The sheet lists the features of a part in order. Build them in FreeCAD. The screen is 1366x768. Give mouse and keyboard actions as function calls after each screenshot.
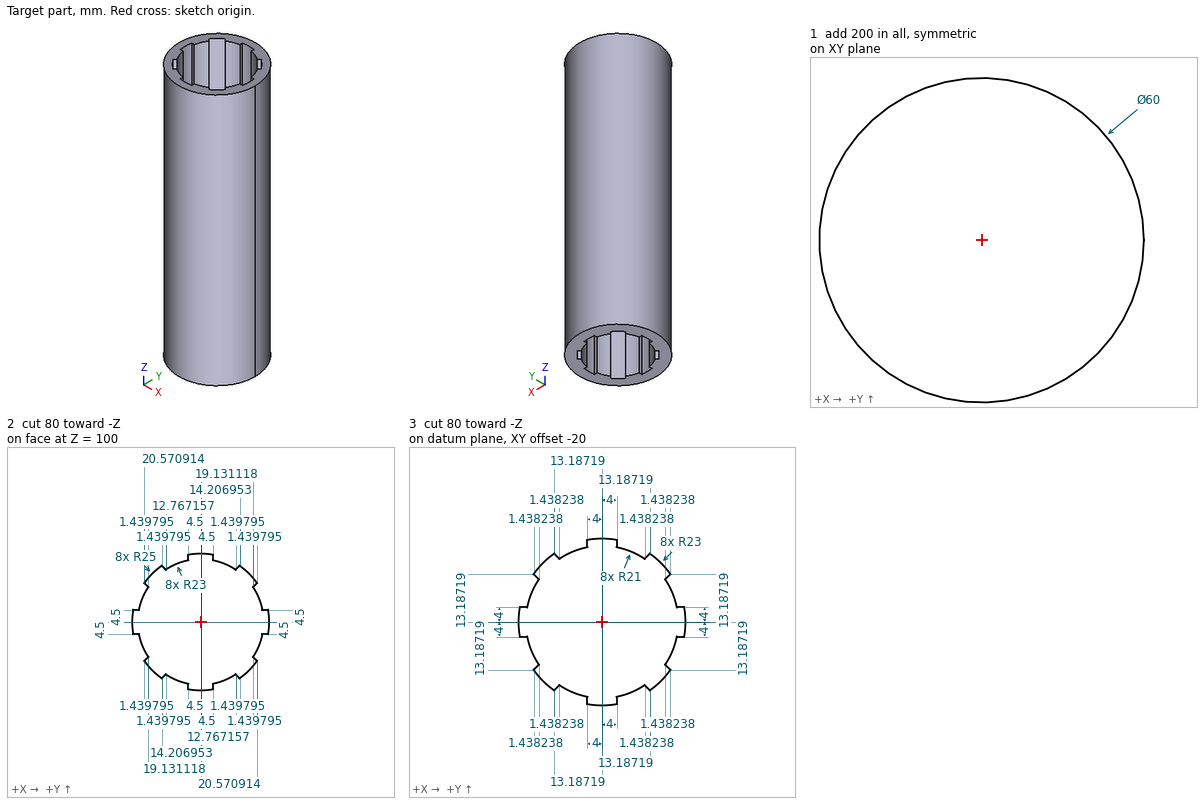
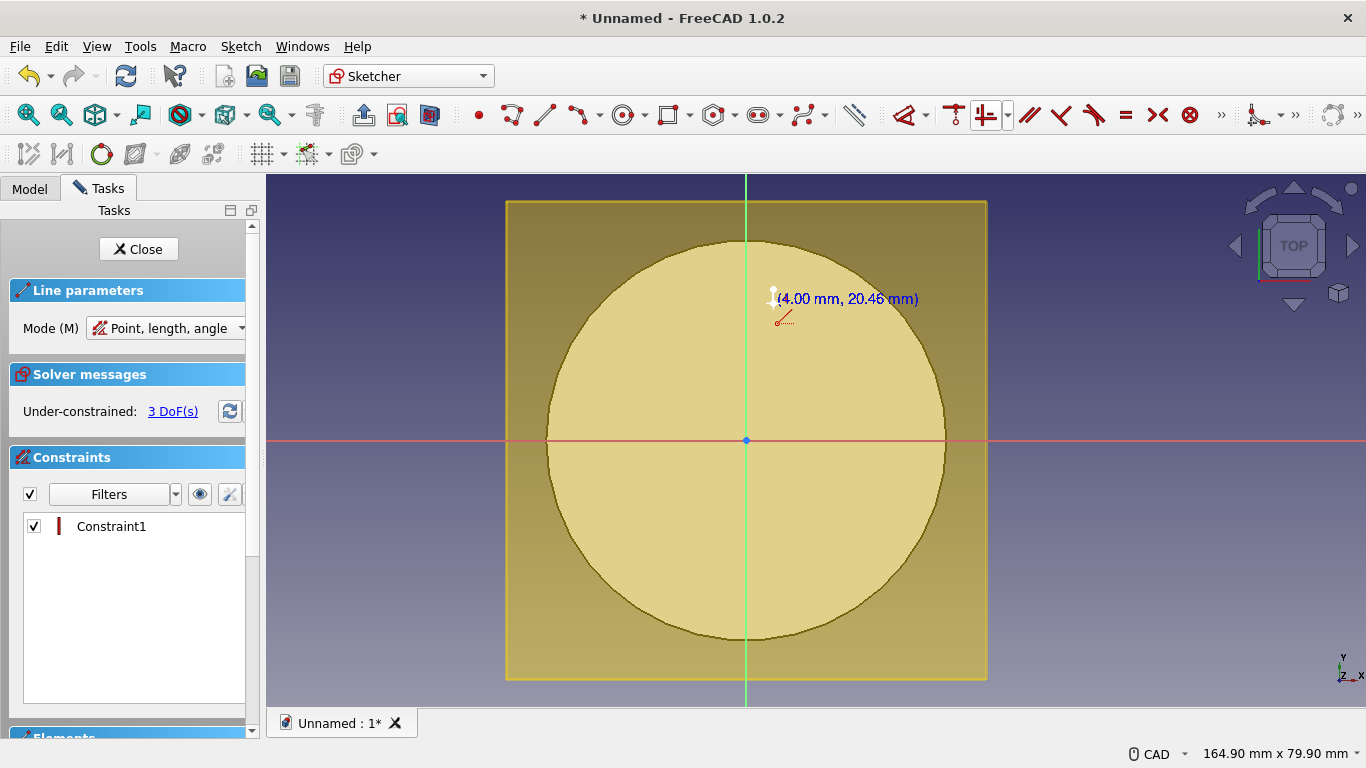
click(825, 324)
click(834, 315)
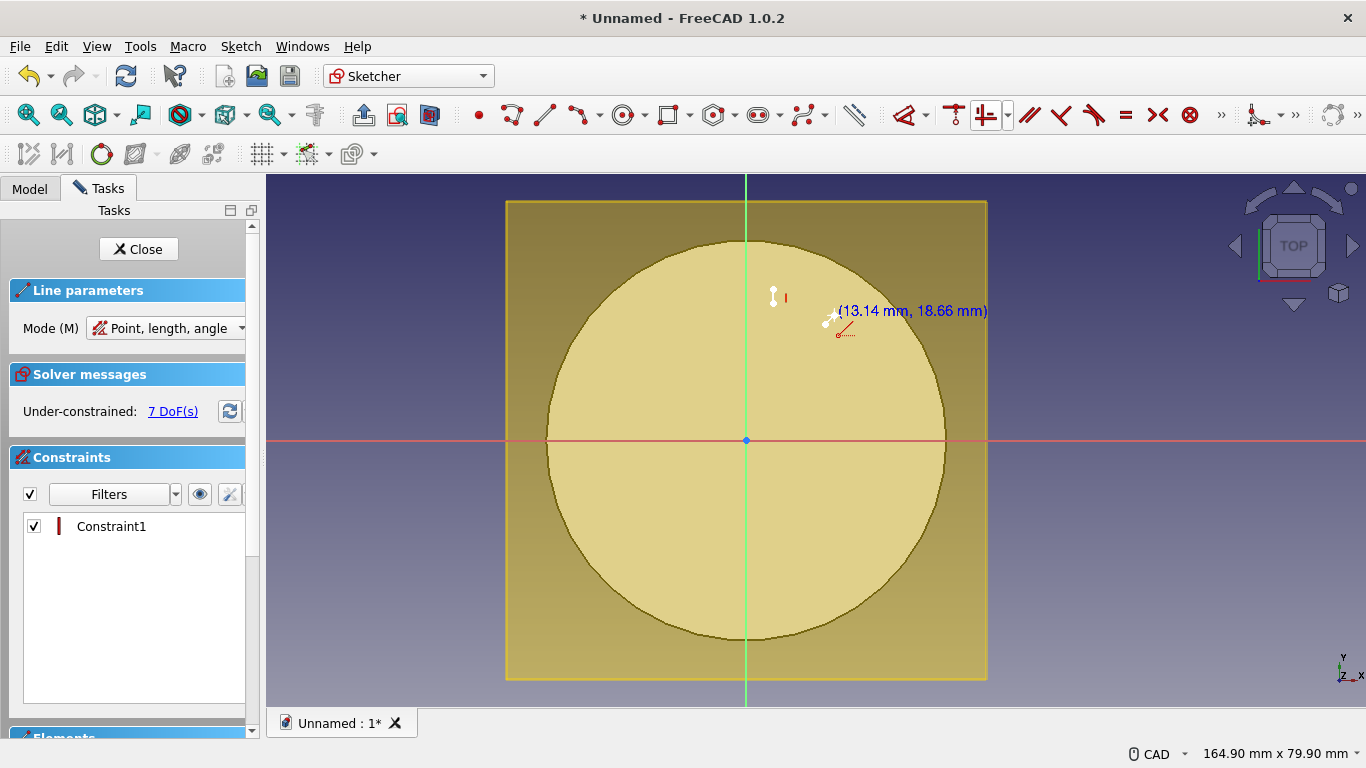
click(872, 353)
click(862, 362)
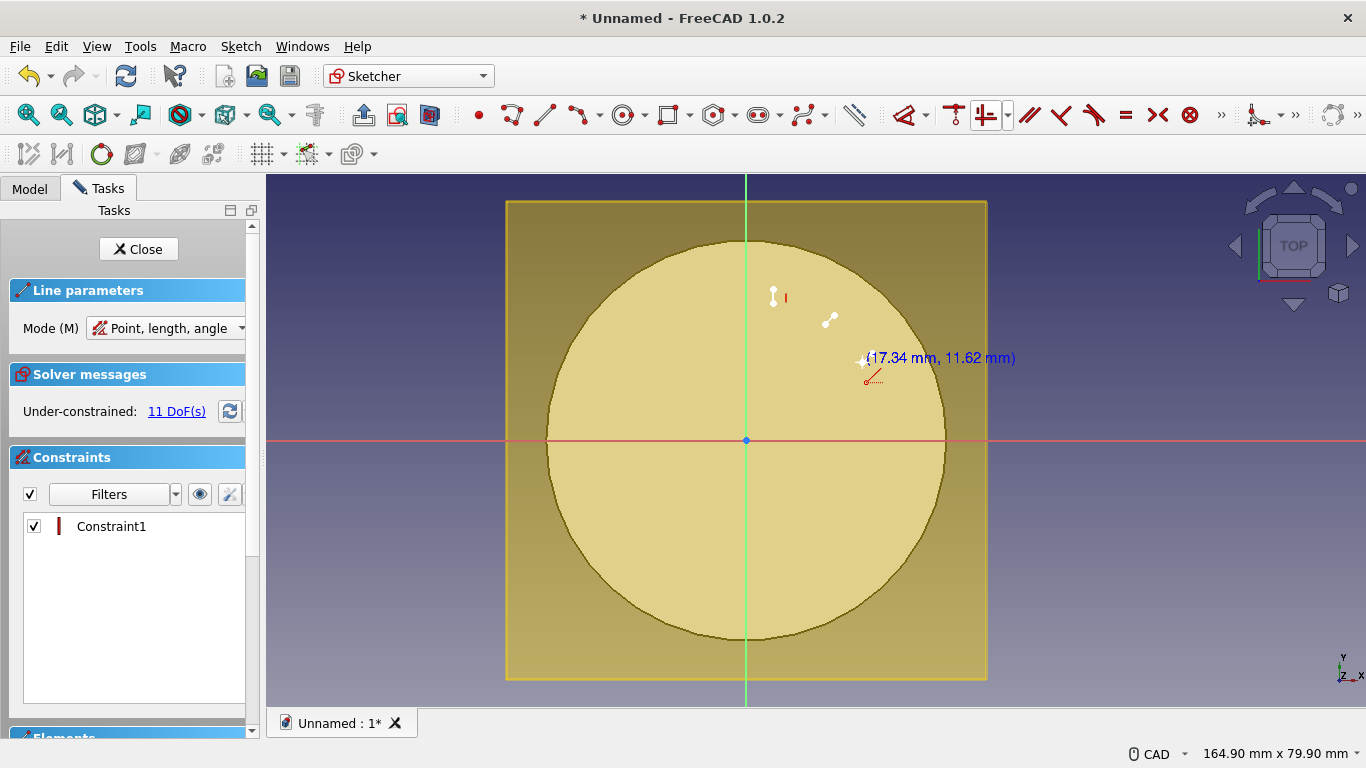
click(884, 414)
click(897, 414)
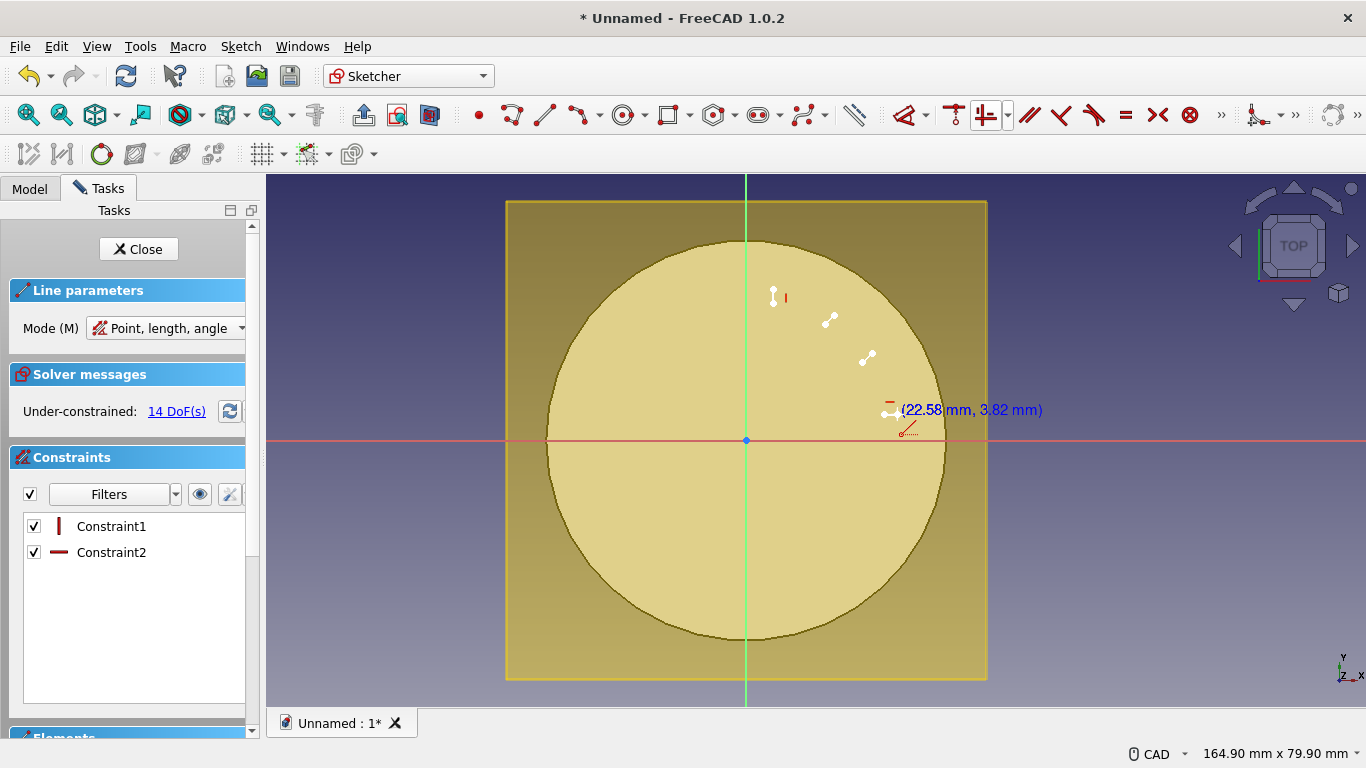
click(897, 467)
click(884, 467)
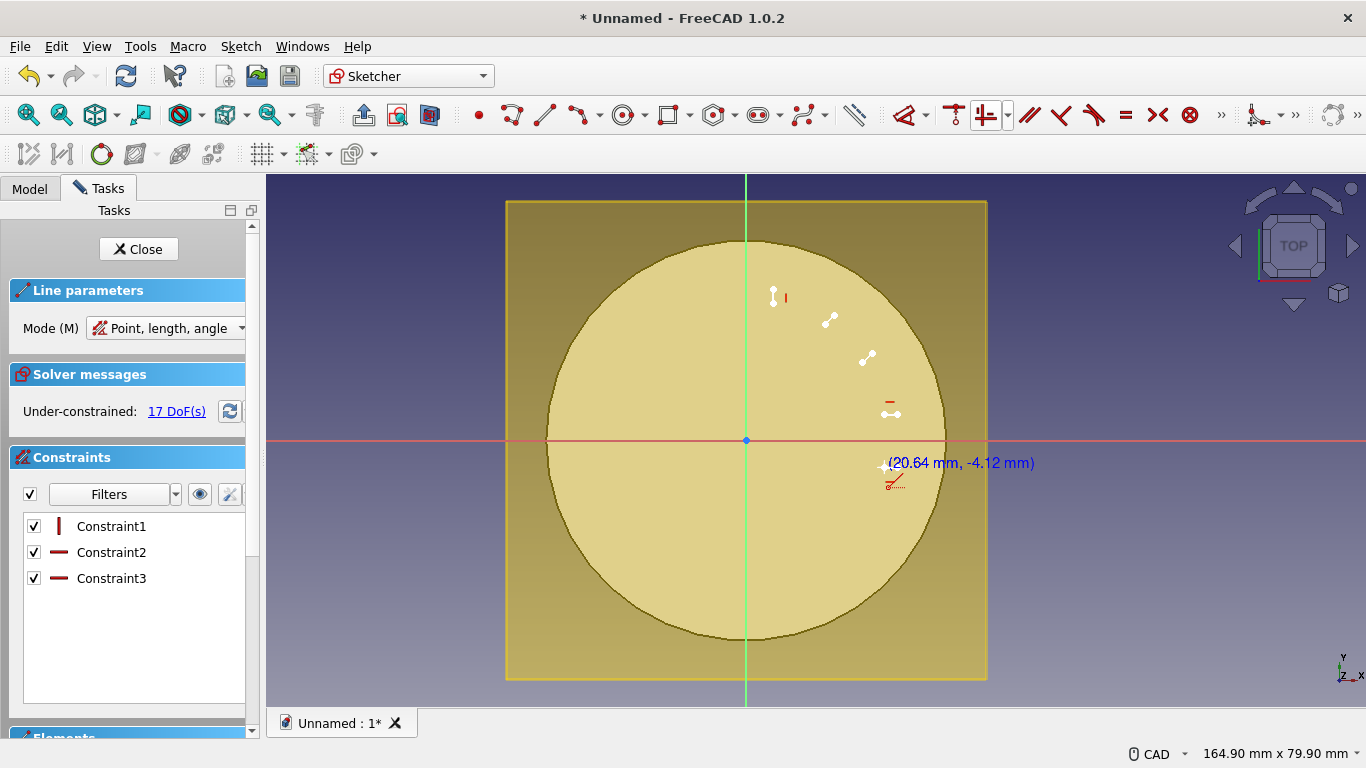
click(862, 519)
click(872, 528)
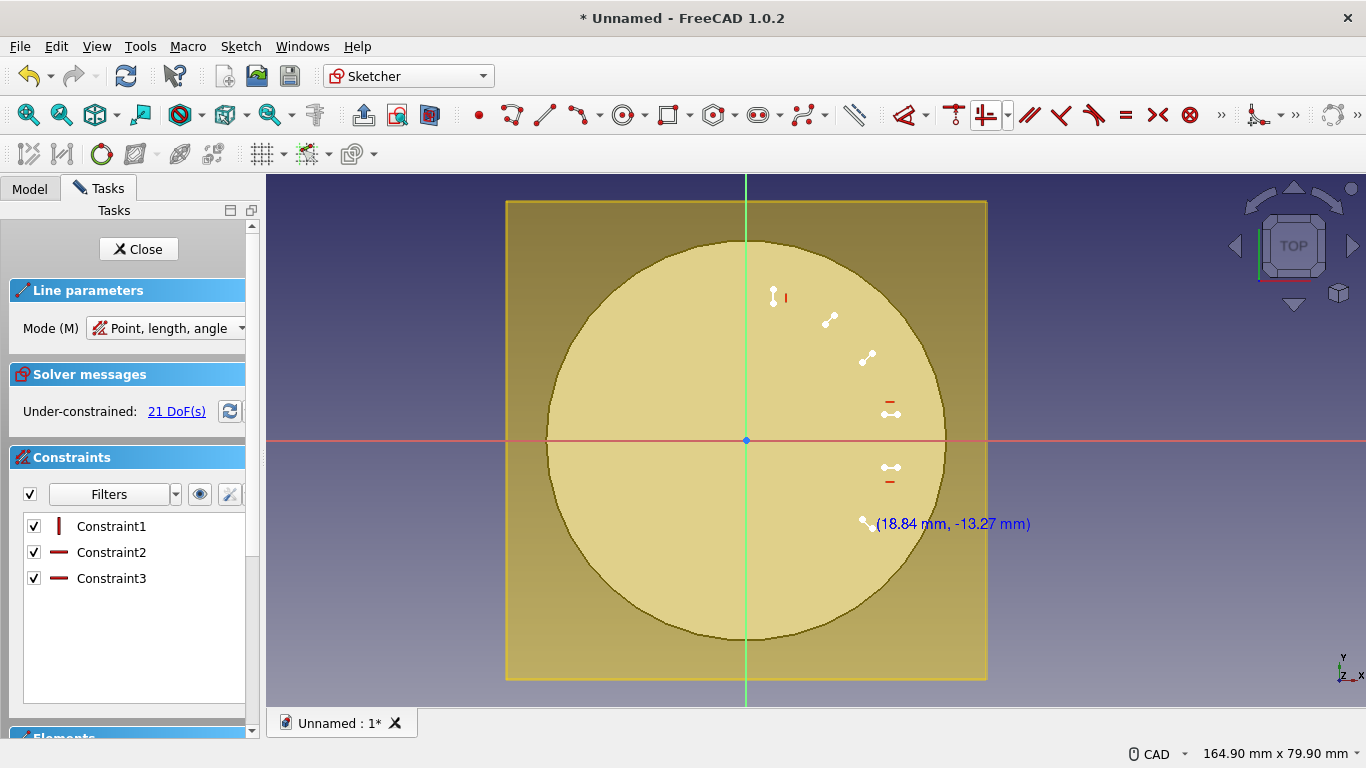
click(834, 566)
click(825, 557)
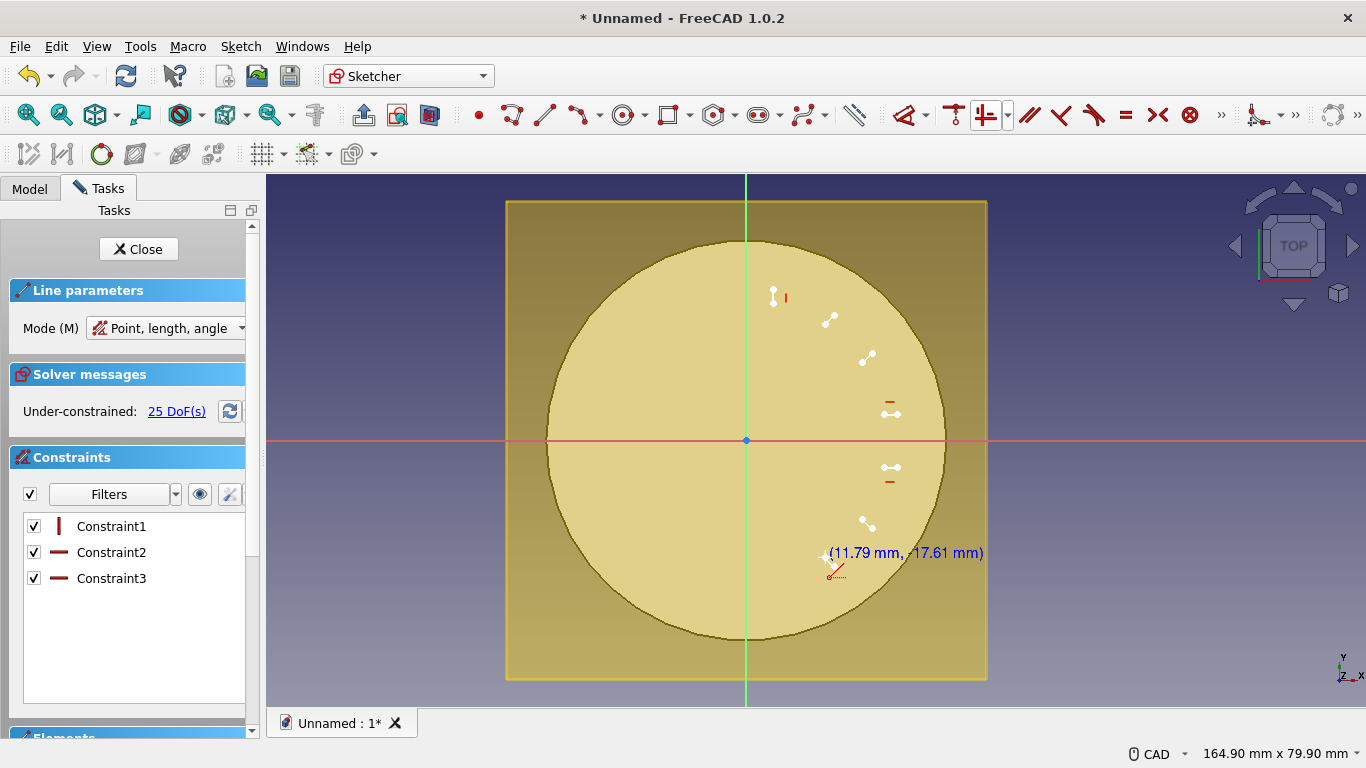
click(773, 578)
click(773, 592)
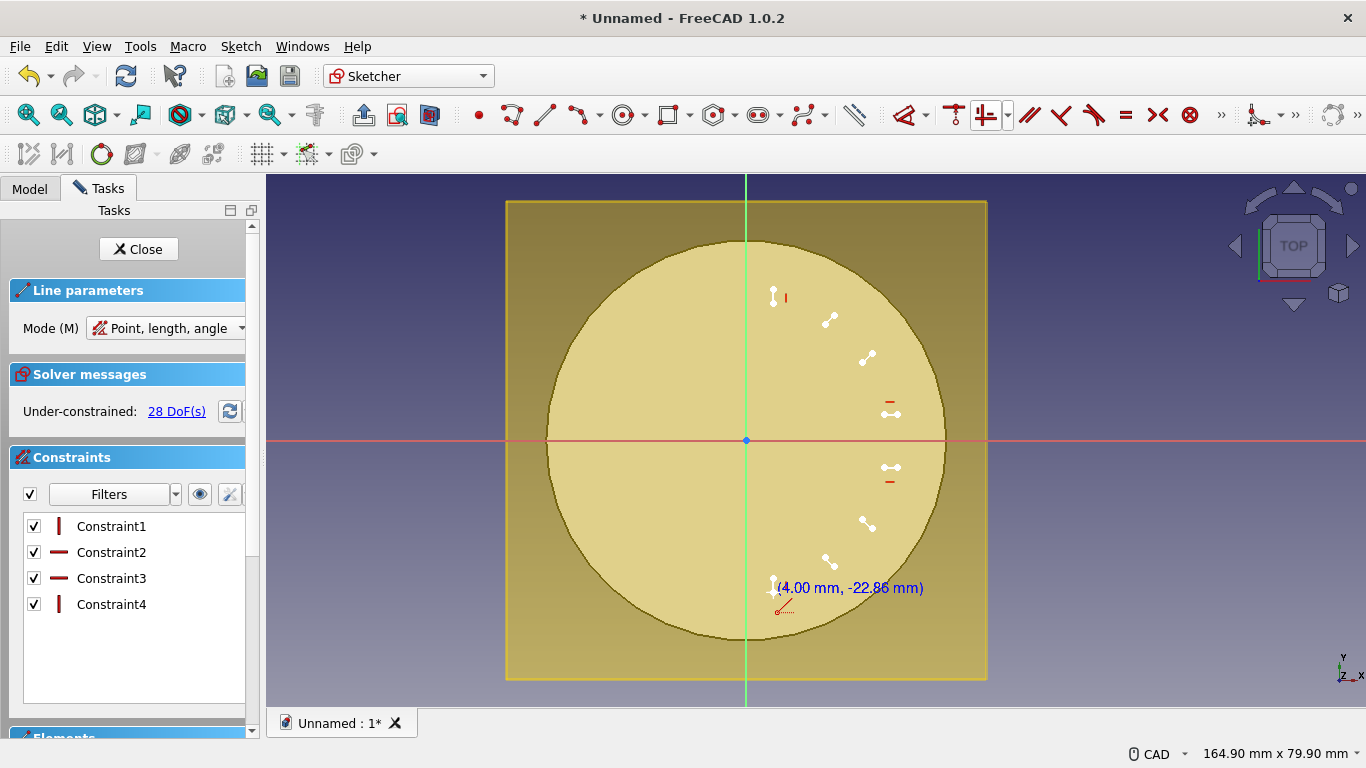
click(720, 592)
click(720, 578)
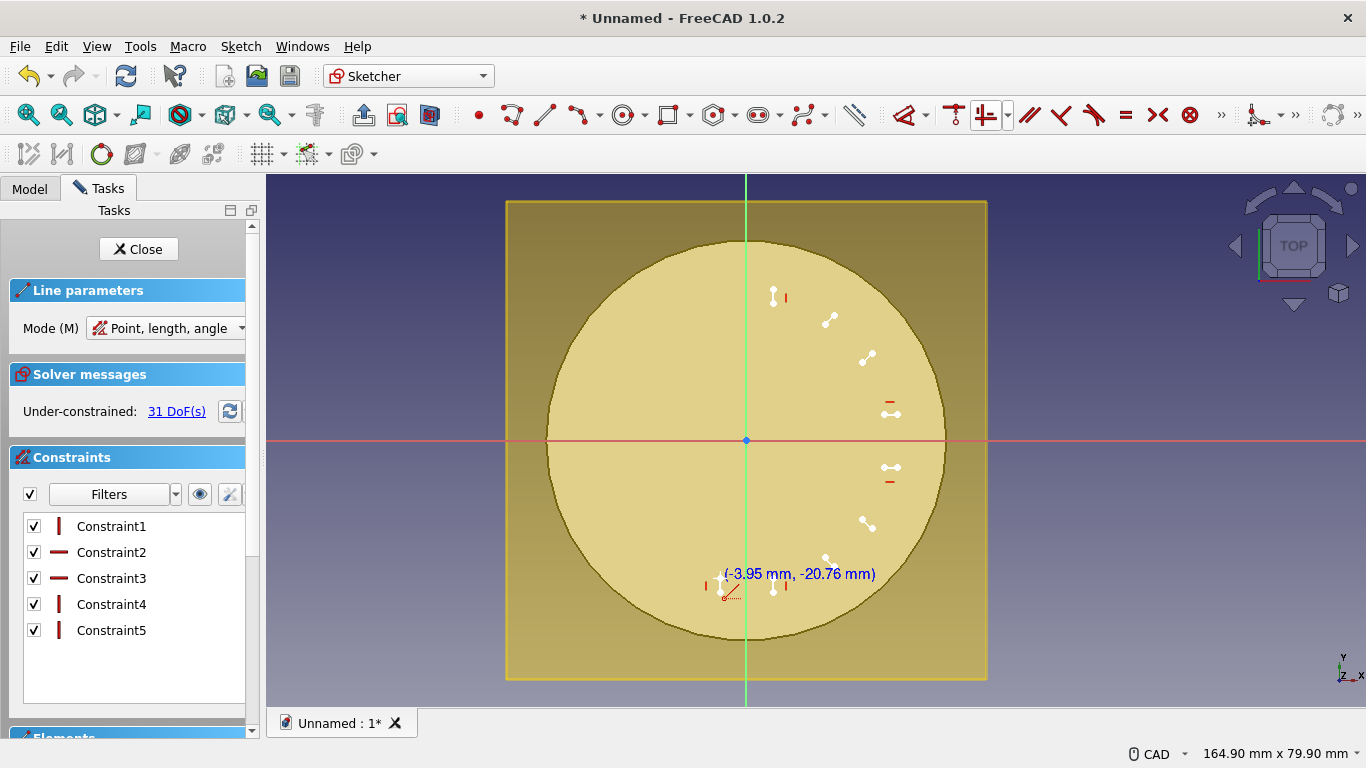
click(668, 557)
click(658, 566)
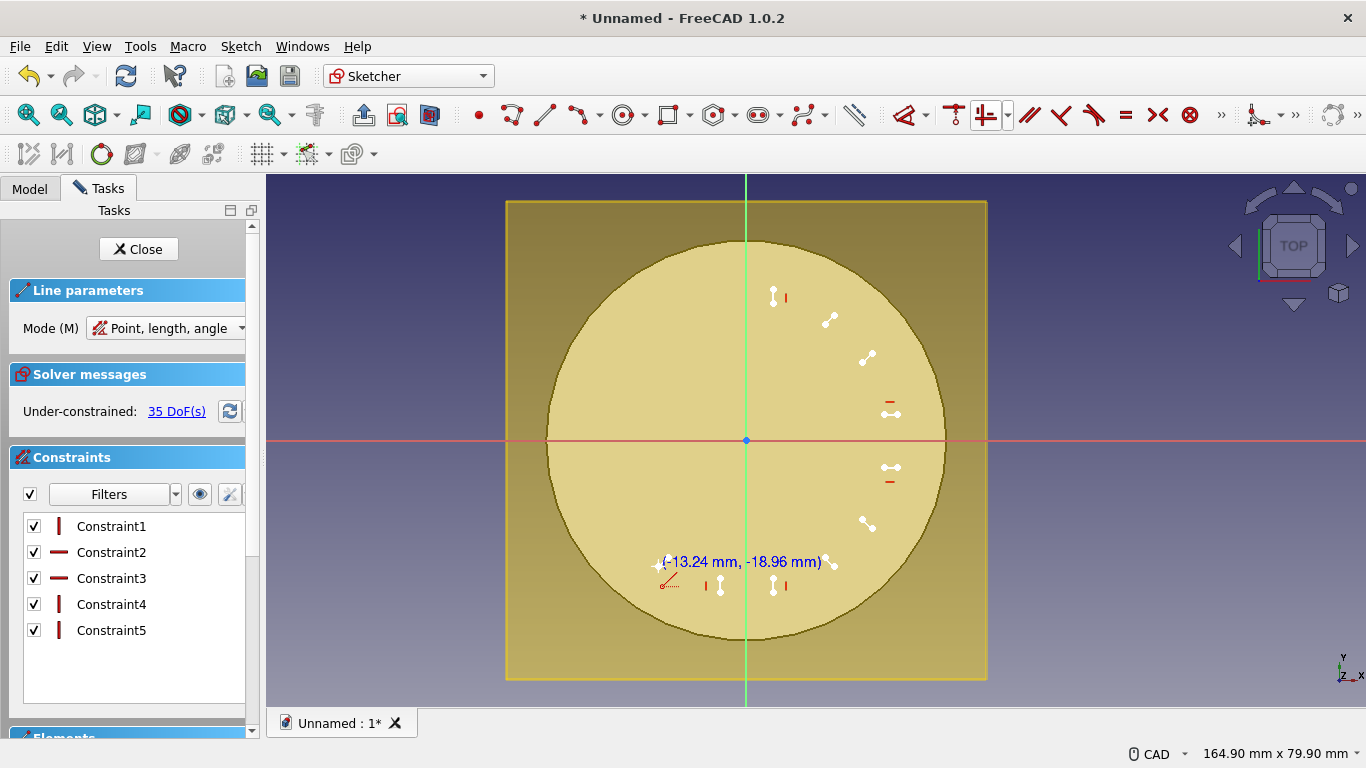
click(621, 528)
click(630, 519)